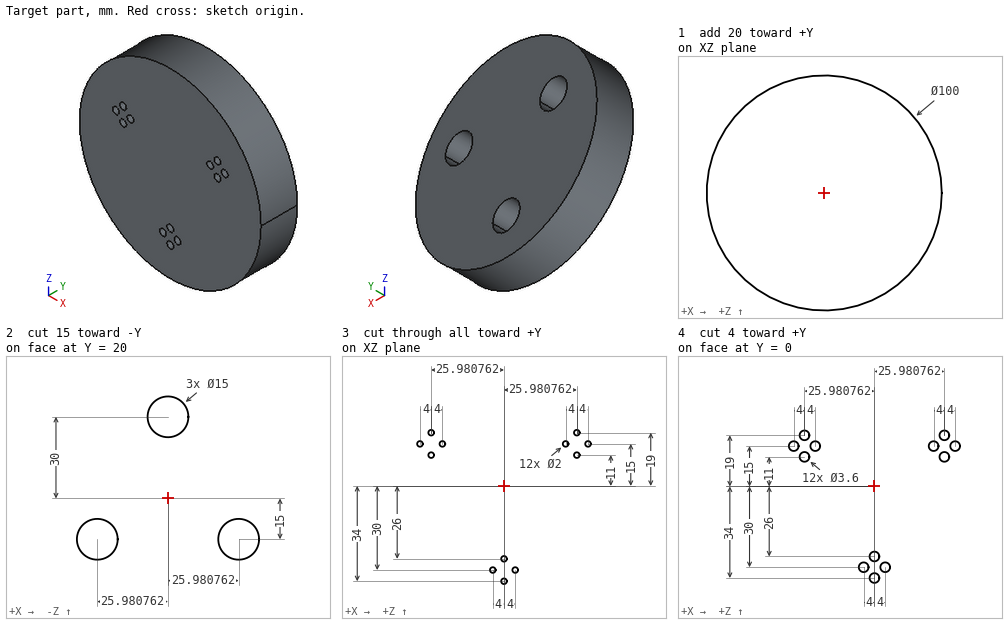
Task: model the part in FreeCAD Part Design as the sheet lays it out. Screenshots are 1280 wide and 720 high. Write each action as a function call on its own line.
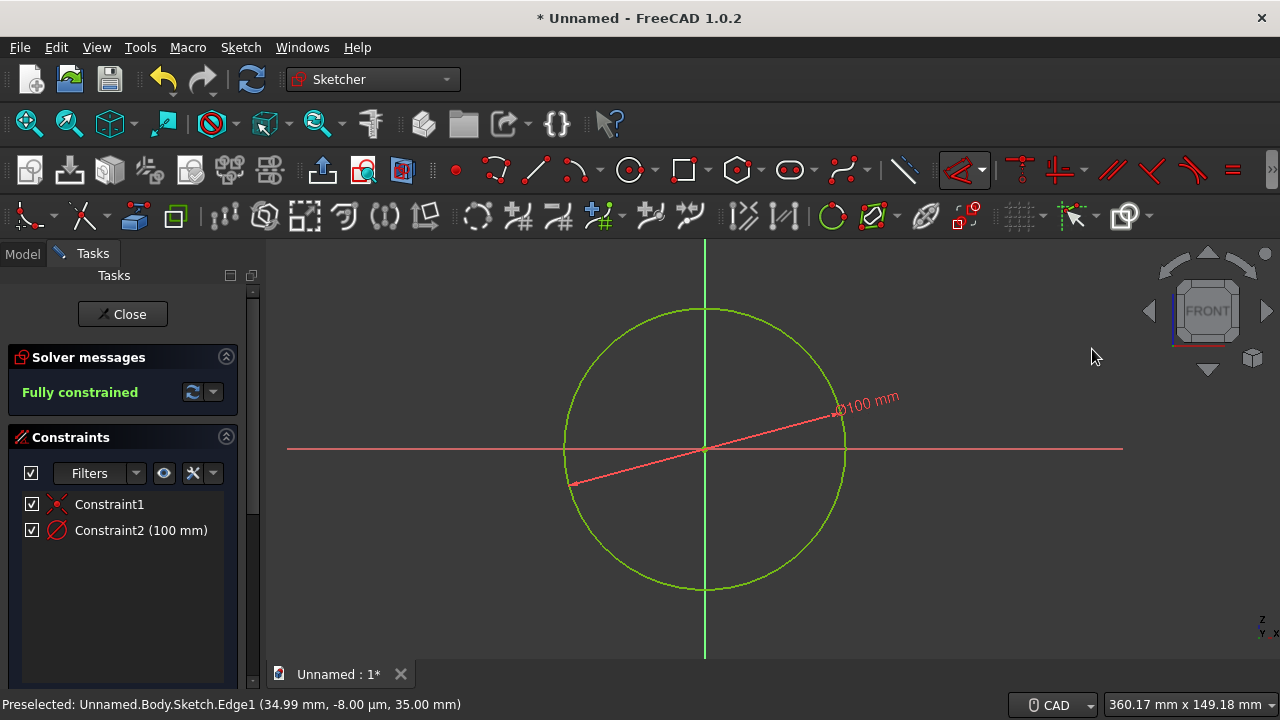
click(123, 314)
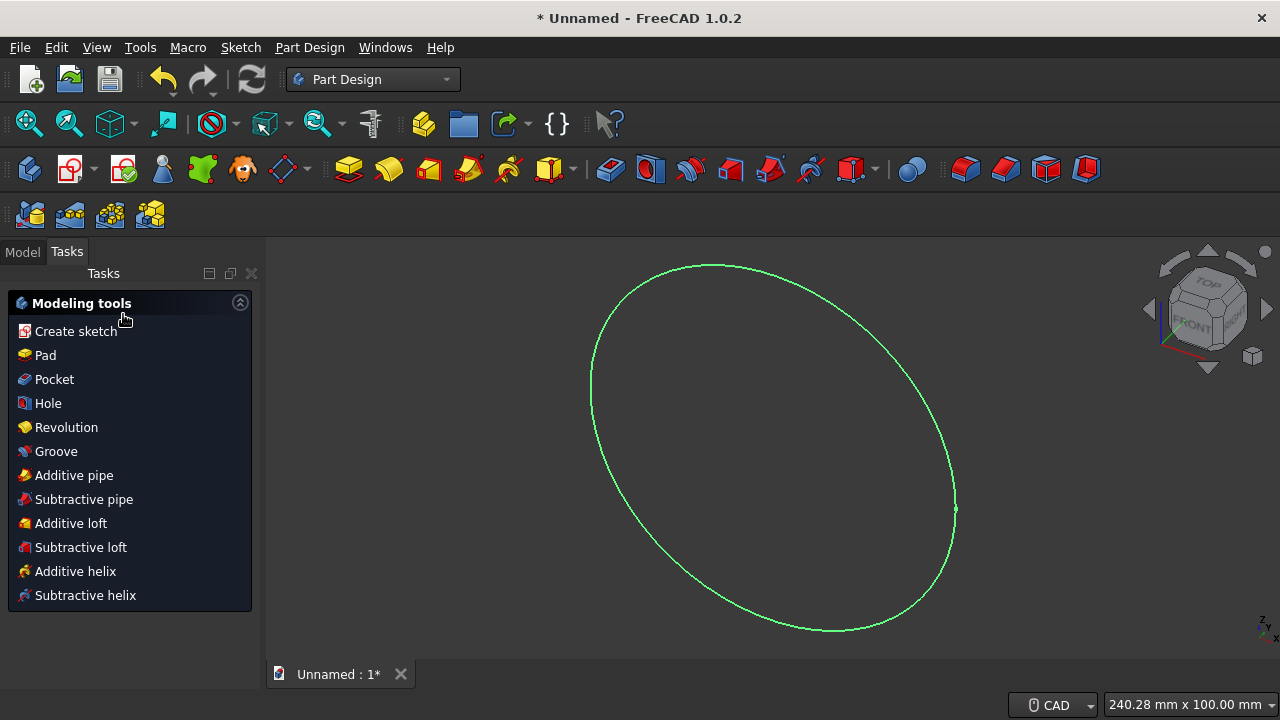
click(350, 170)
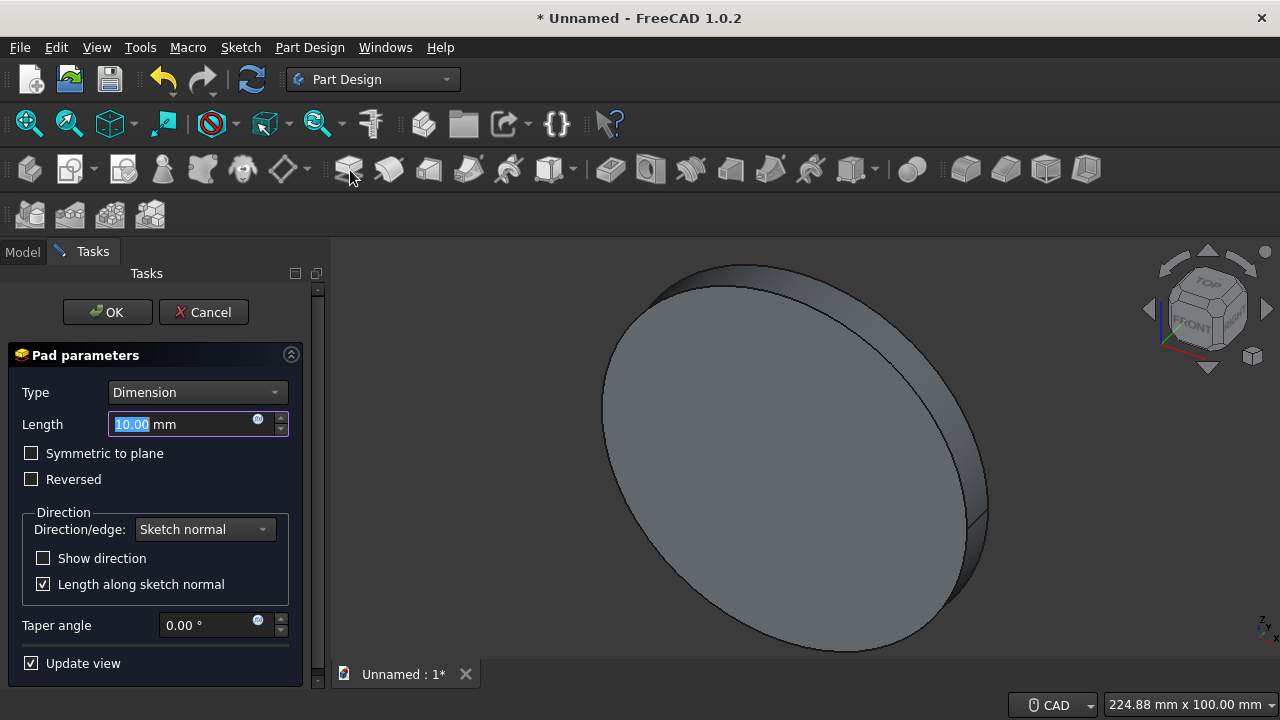
text(20)
key(Tab)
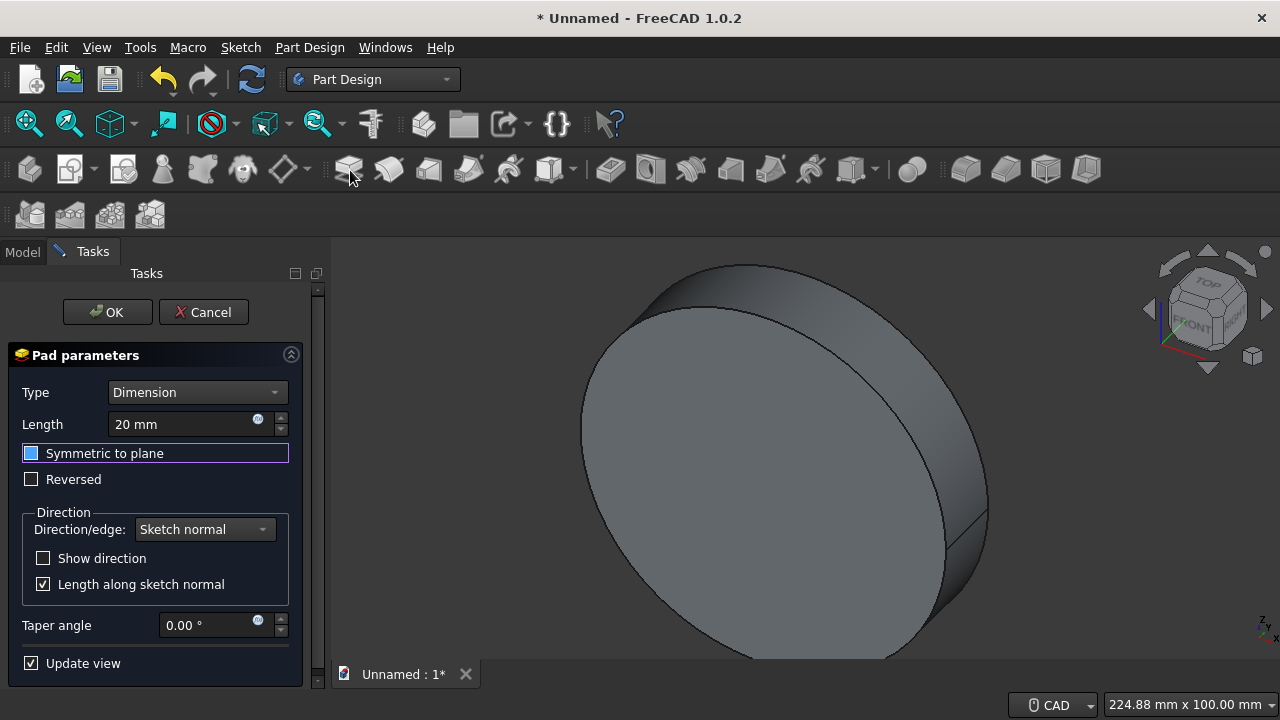
click(30, 479)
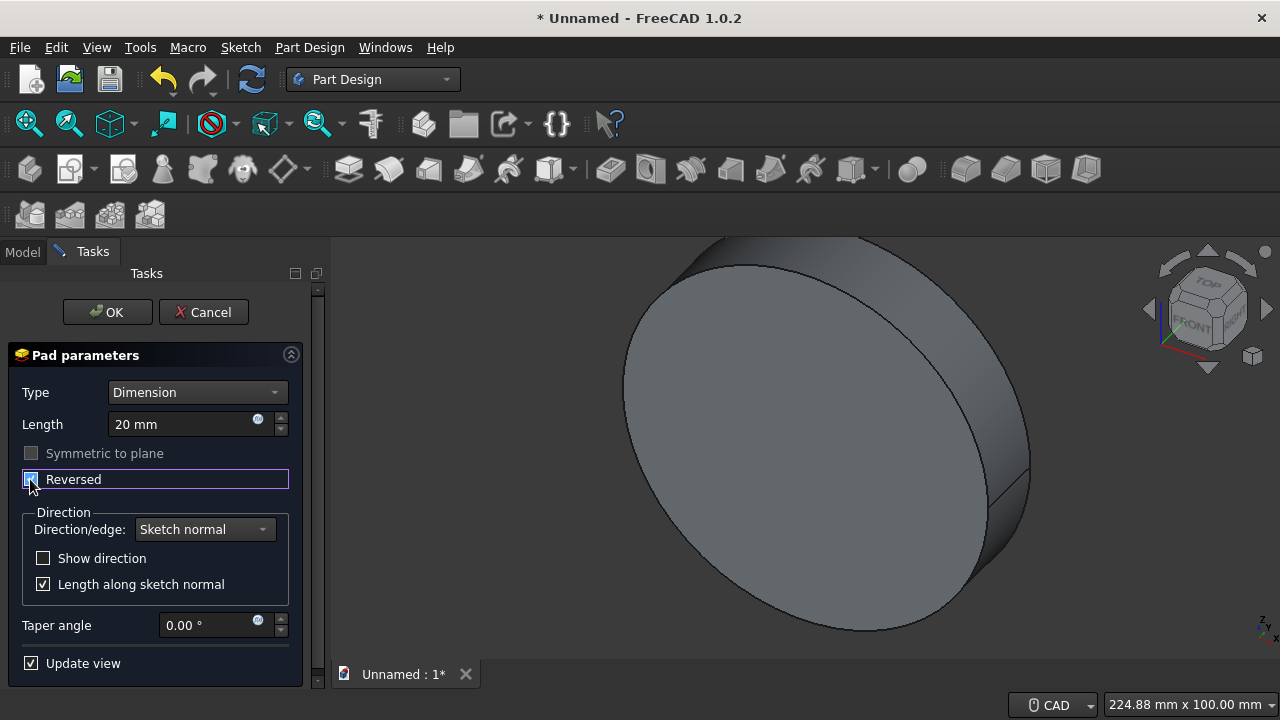
click(108, 312)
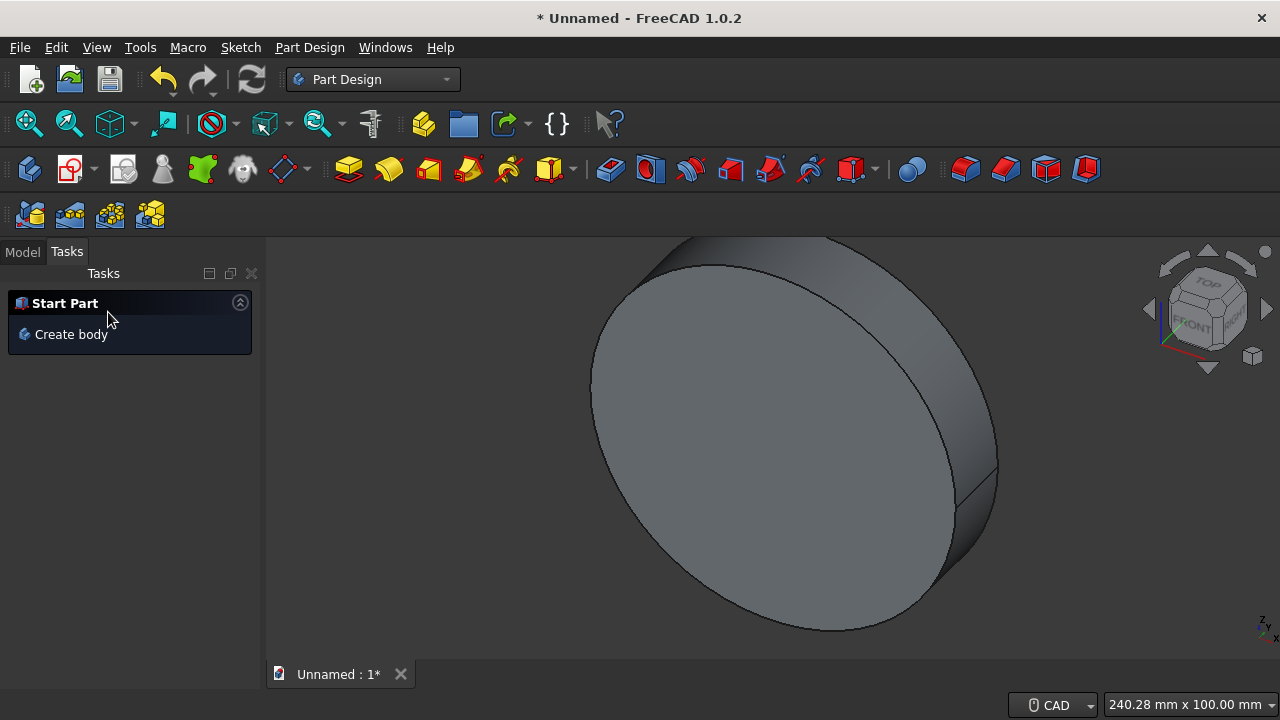
click(30, 124)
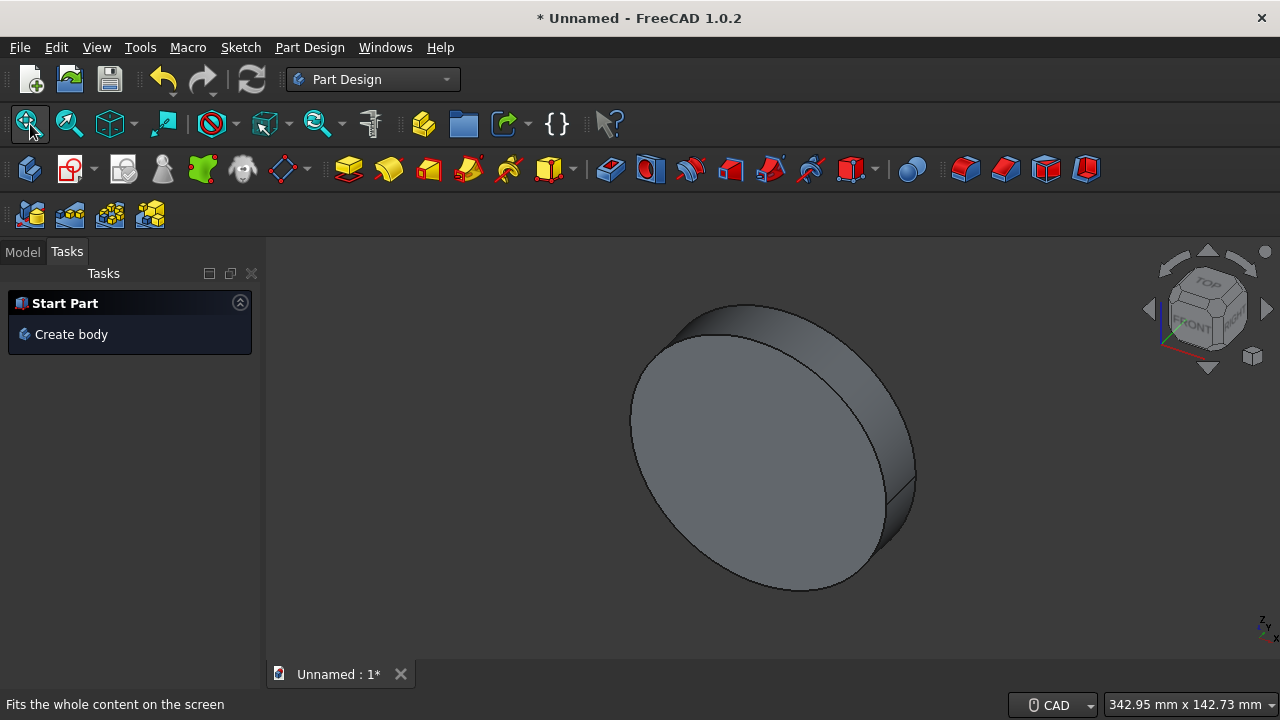
key(4)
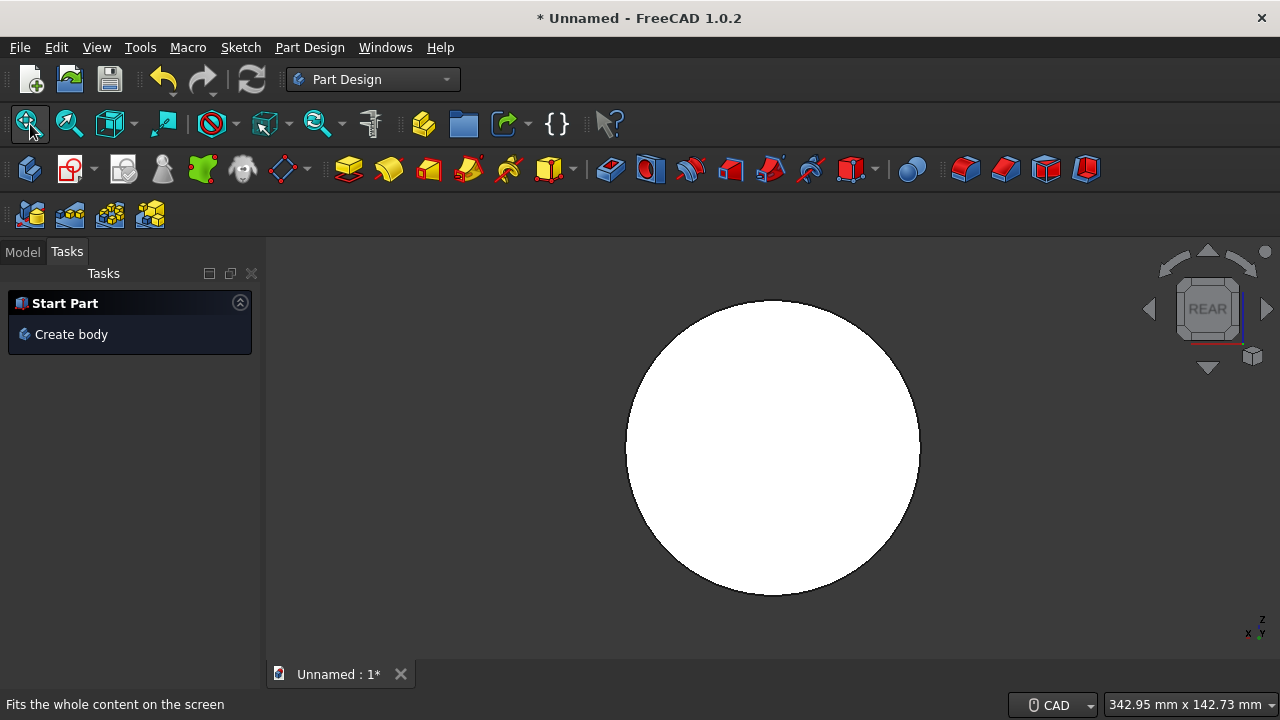
click(773, 447)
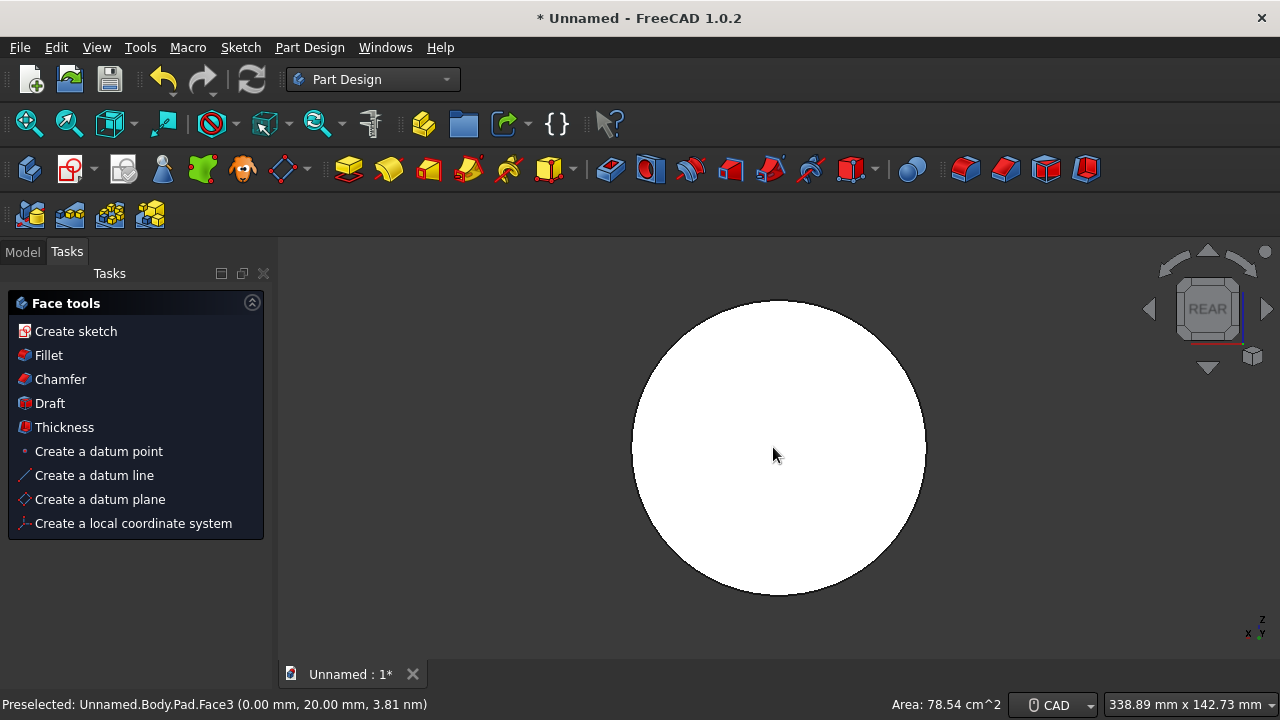
click(70, 170)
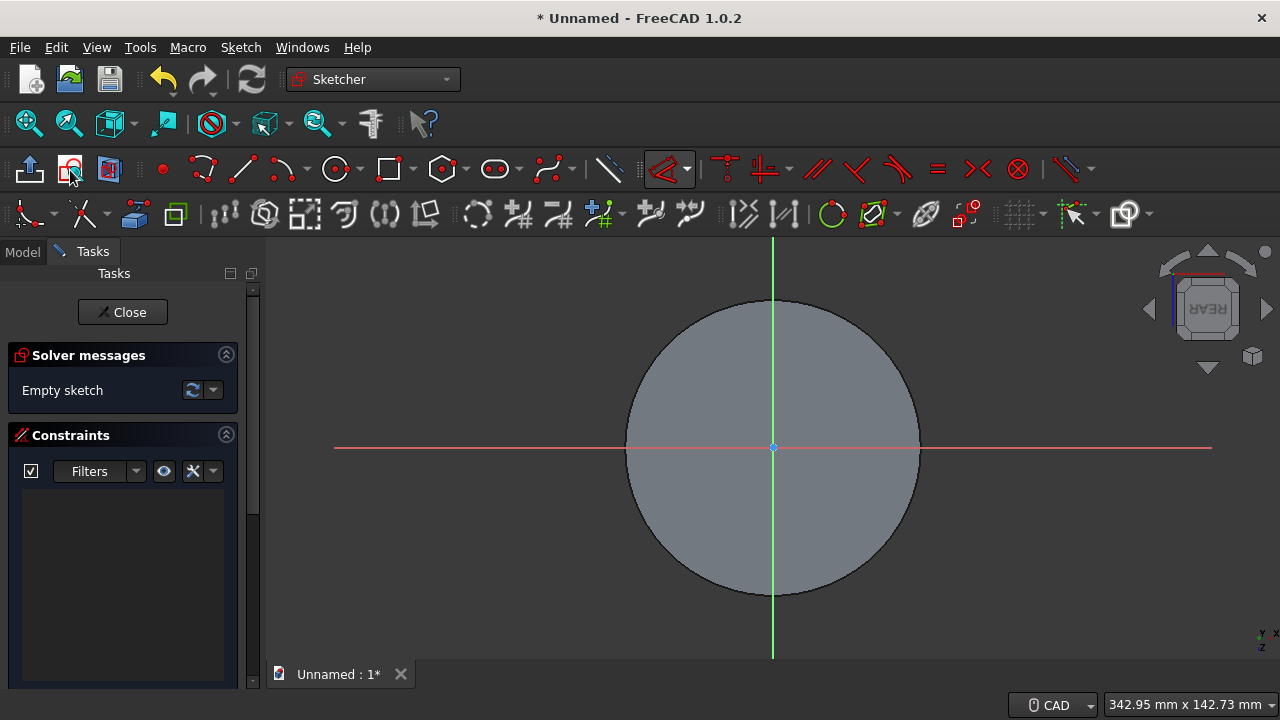
scroll(912, 381, up, 2)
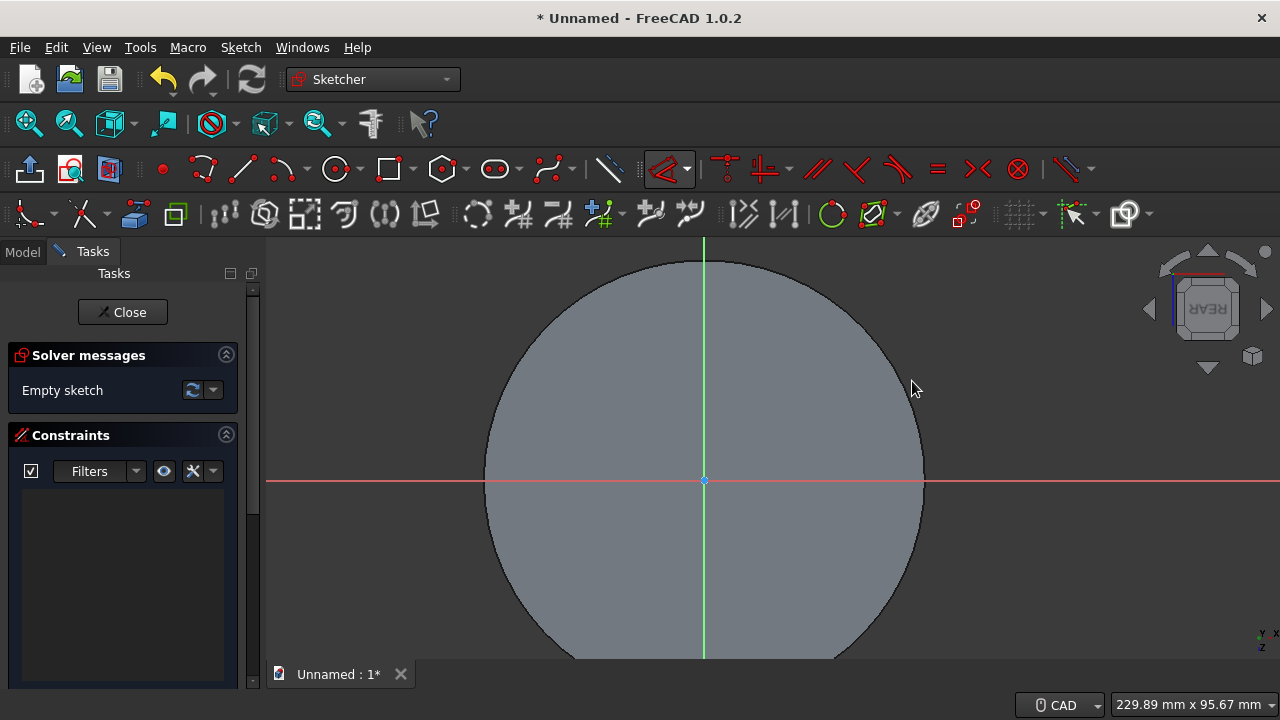
click(336, 170)